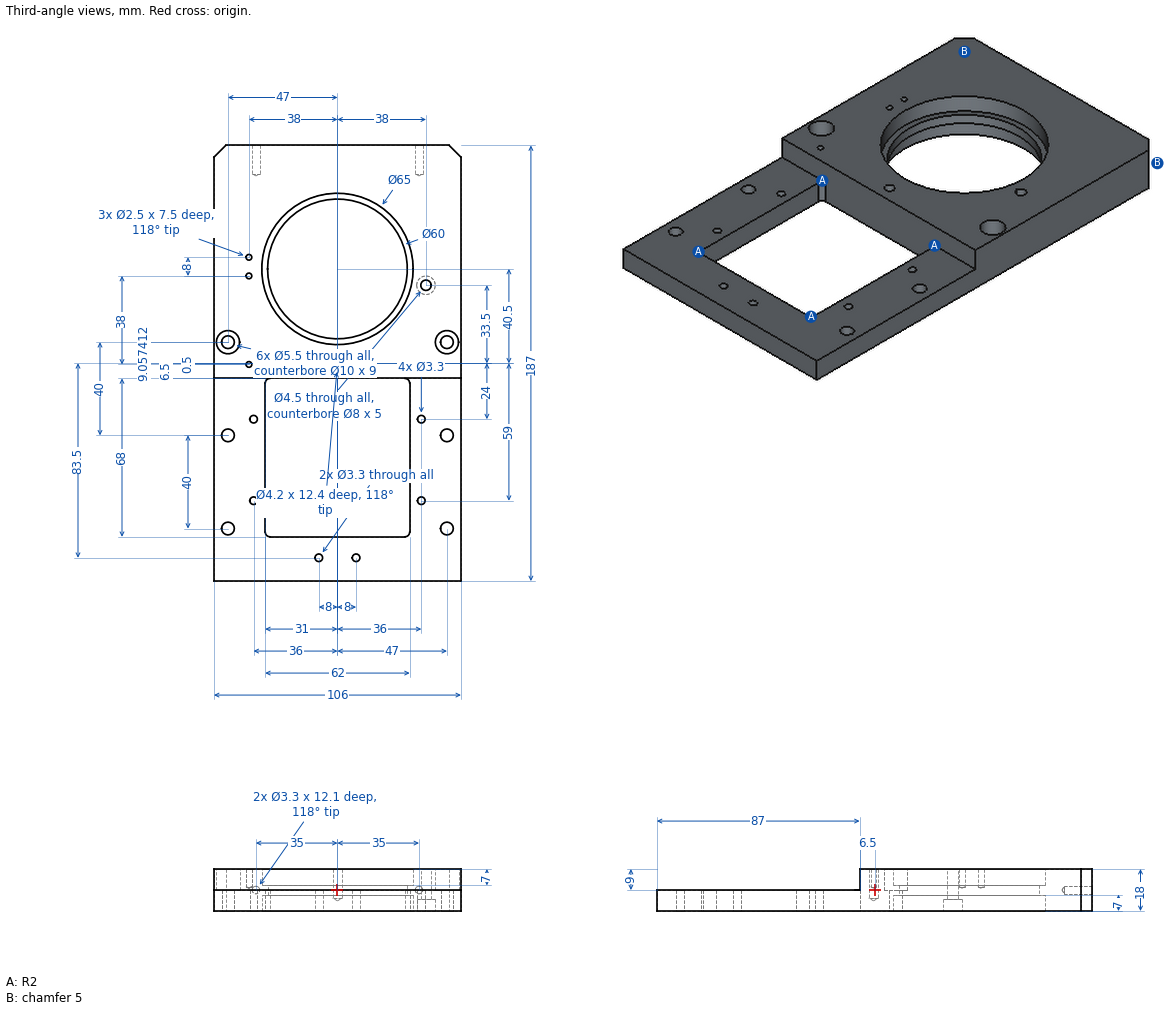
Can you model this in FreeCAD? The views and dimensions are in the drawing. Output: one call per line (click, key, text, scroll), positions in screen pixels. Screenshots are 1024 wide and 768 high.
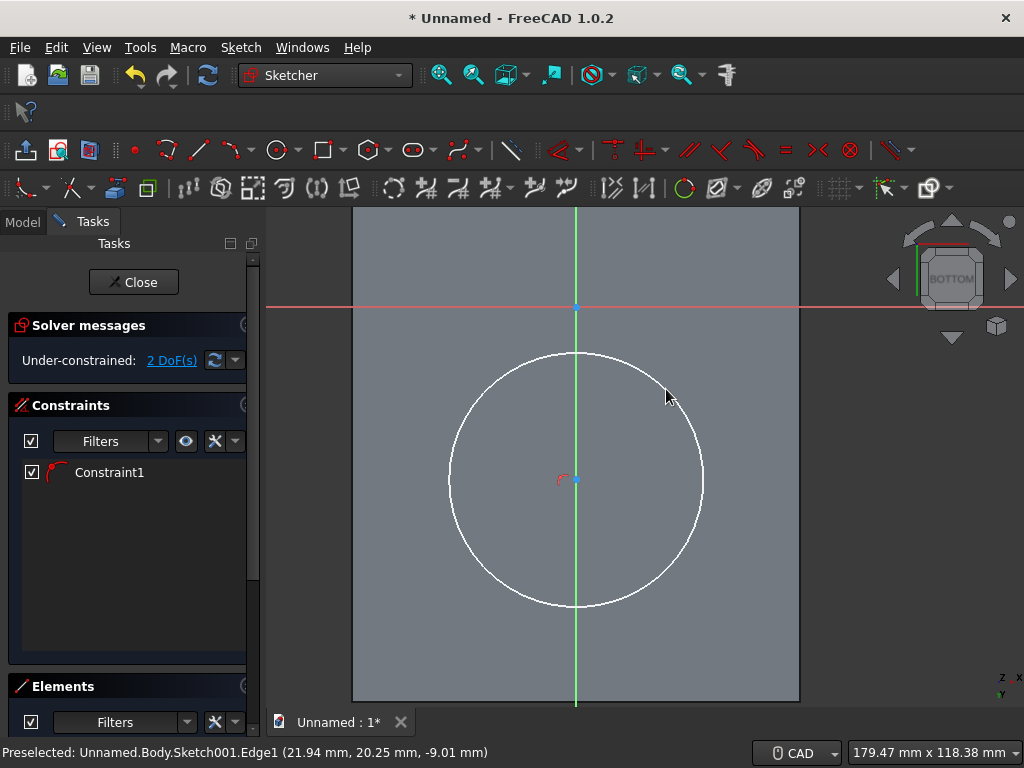
click(558, 150)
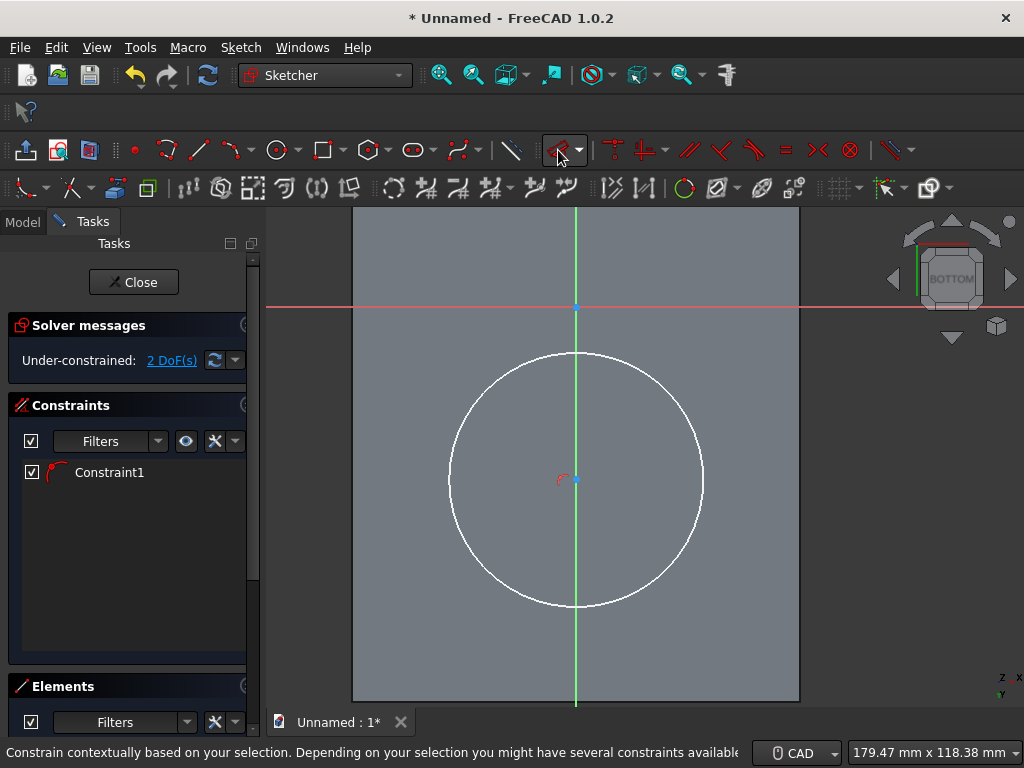
click(666, 390)
click(689, 367)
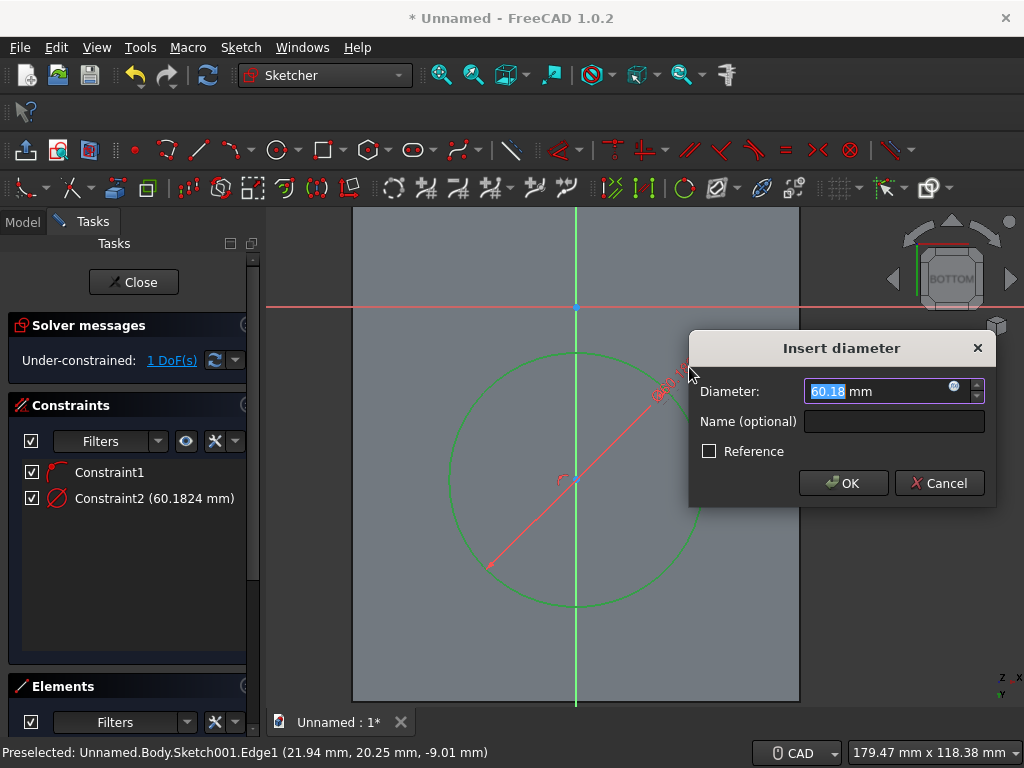
text(60)
key(Return)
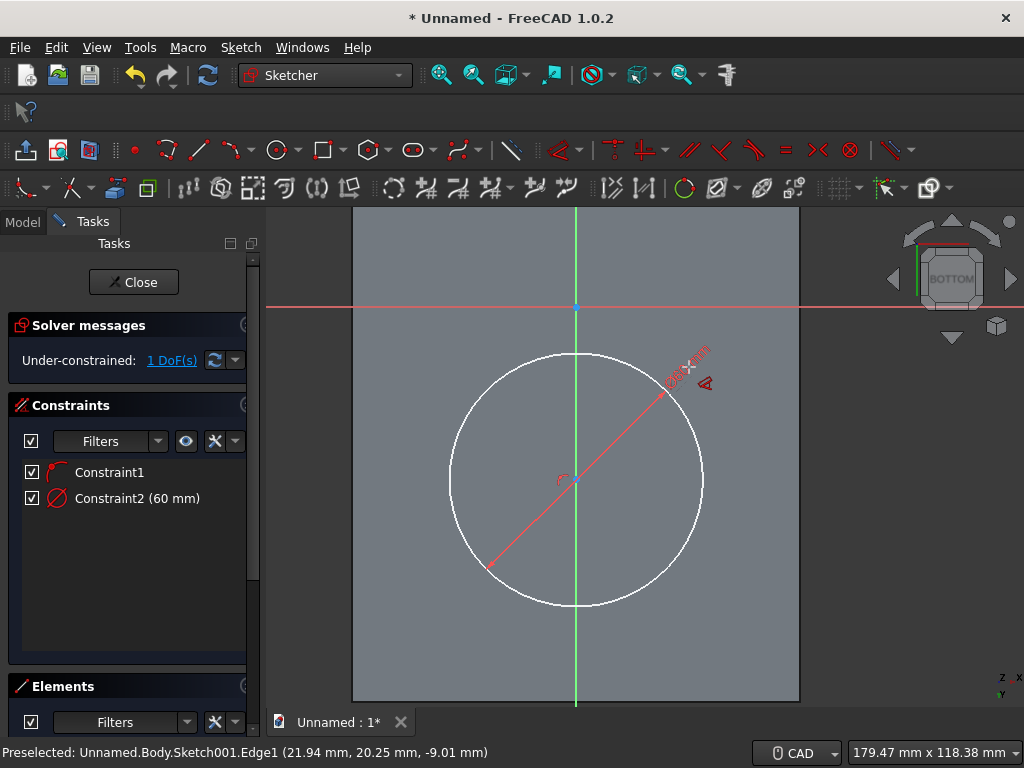
click(576, 480)
click(610, 394)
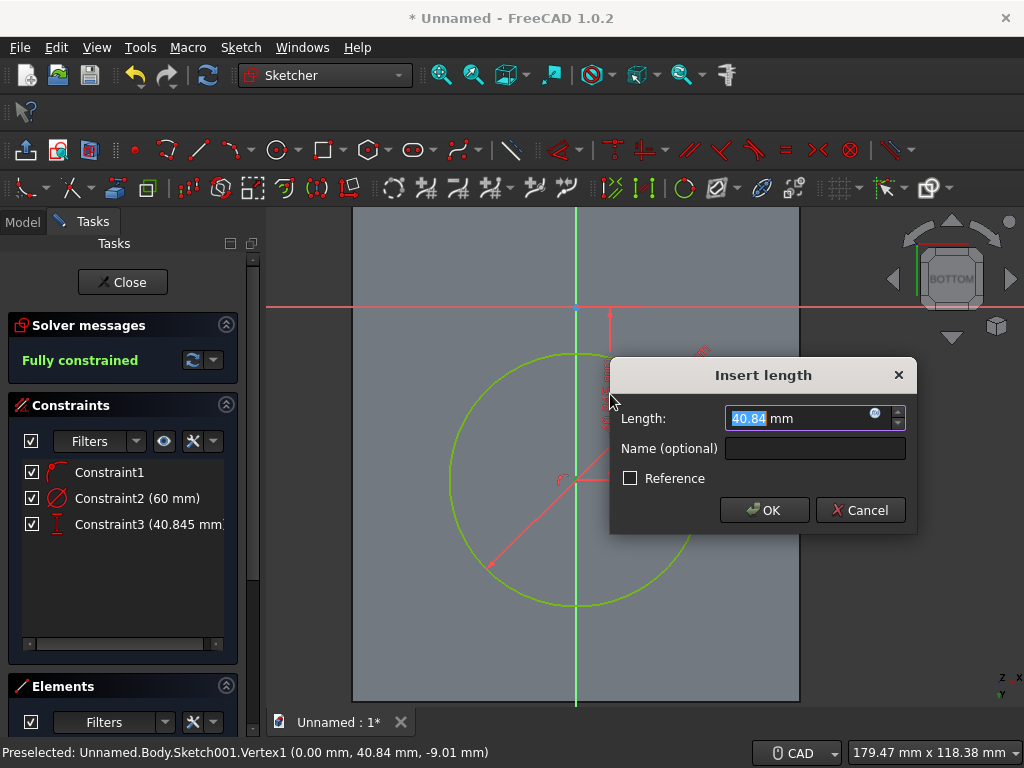
text(40.5)
key(Return)
key(Escape)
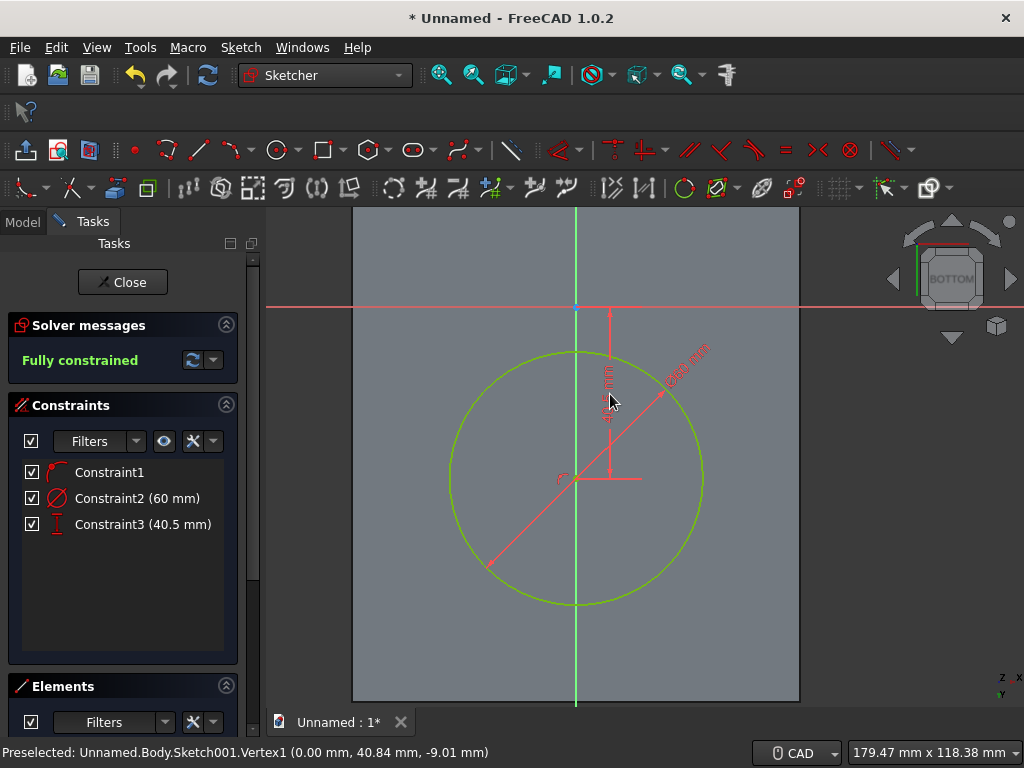
click(123, 282)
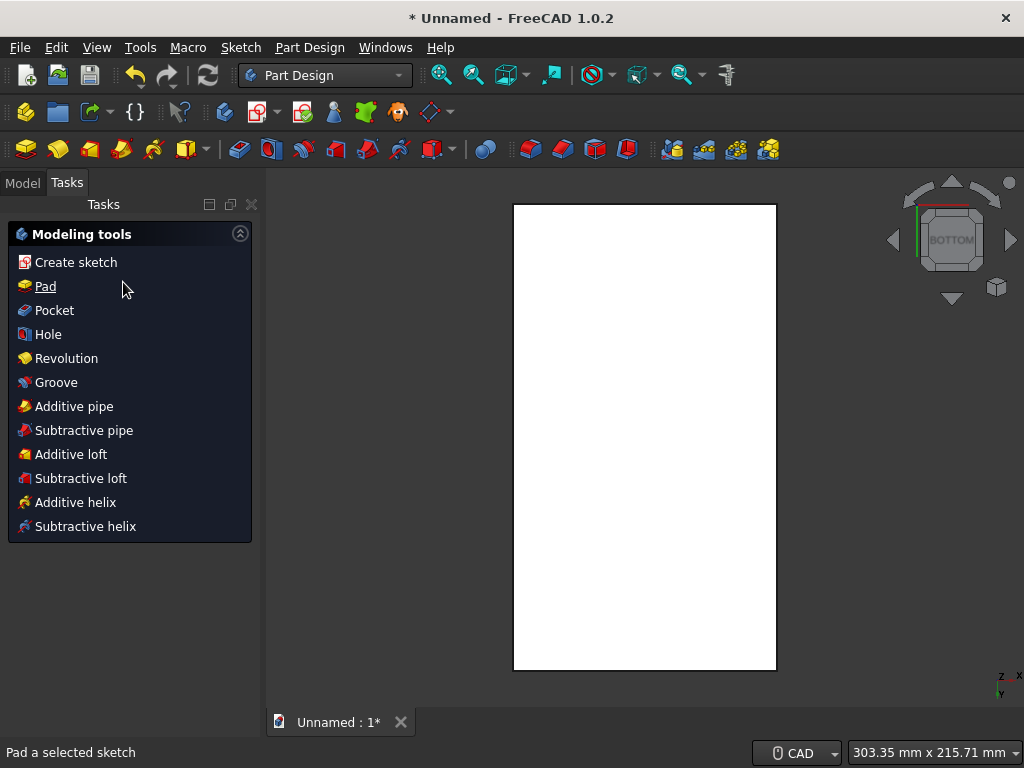
click(240, 150)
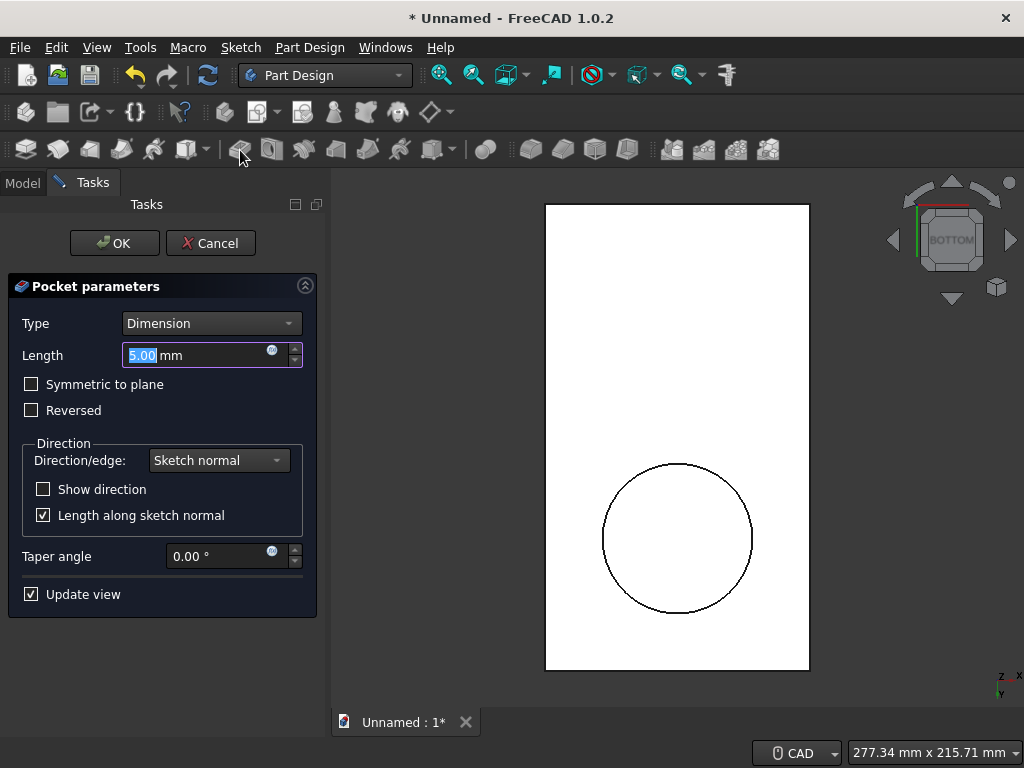
click(212, 324)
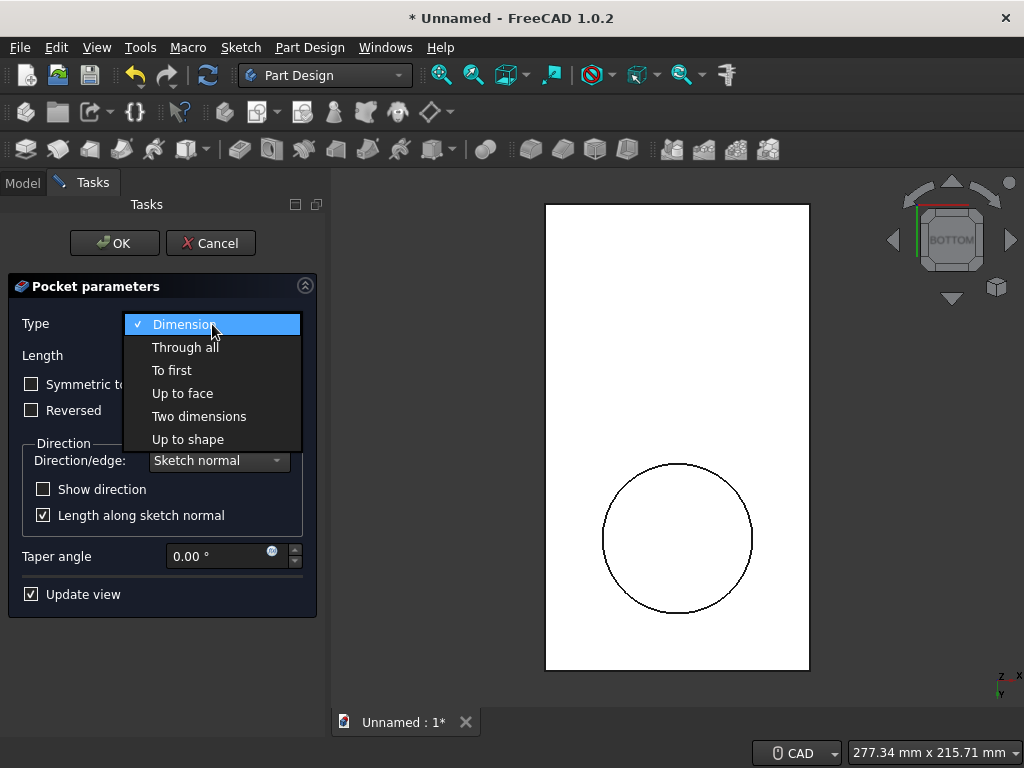
click(212, 348)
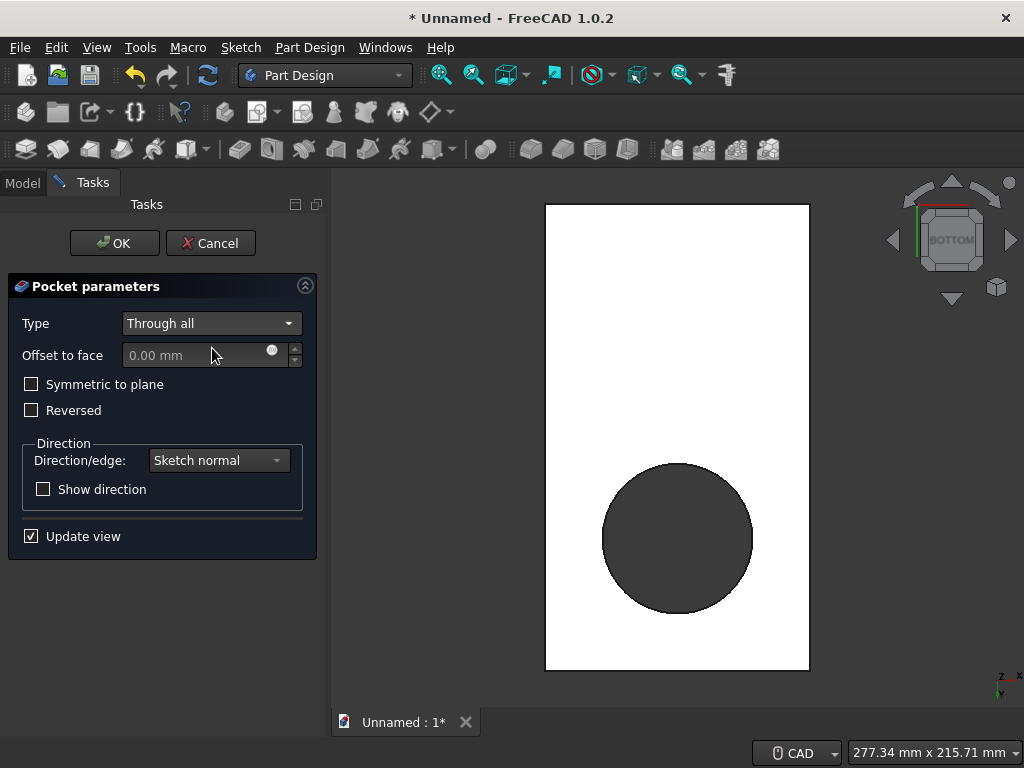
click(115, 243)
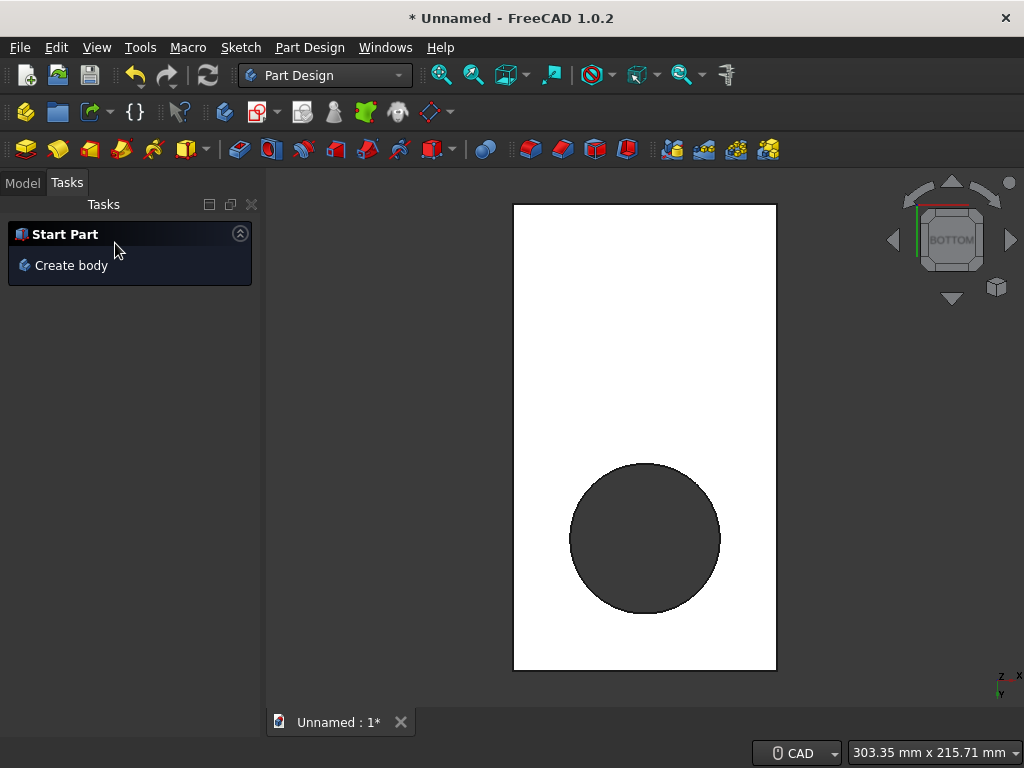
key(0)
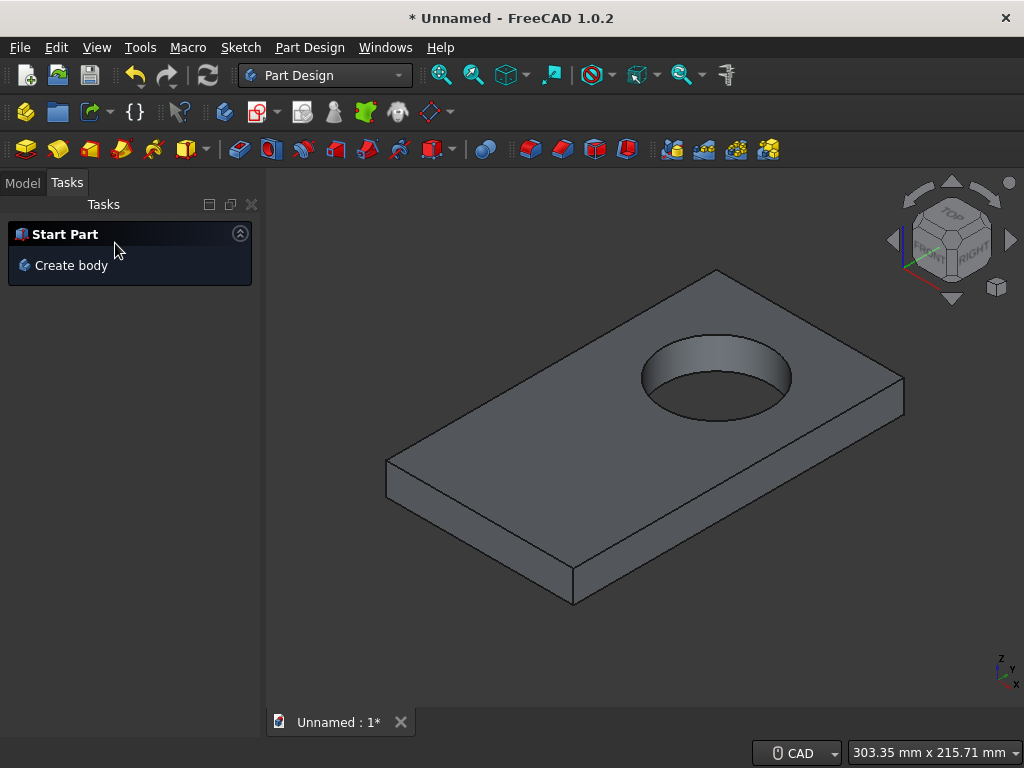
click(551, 473)